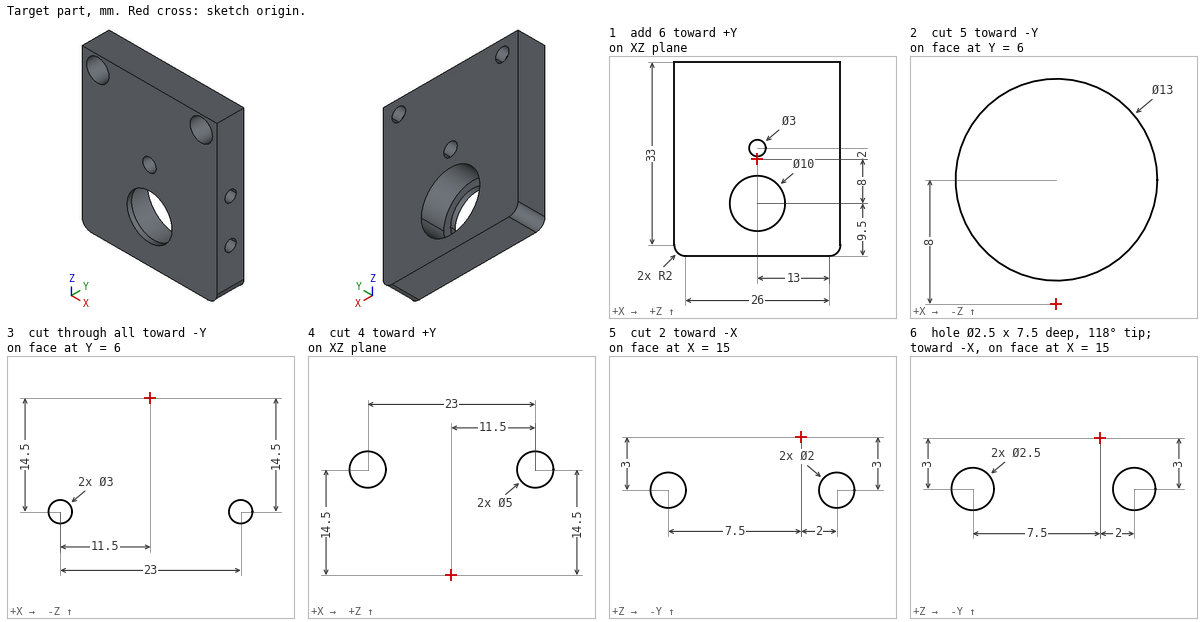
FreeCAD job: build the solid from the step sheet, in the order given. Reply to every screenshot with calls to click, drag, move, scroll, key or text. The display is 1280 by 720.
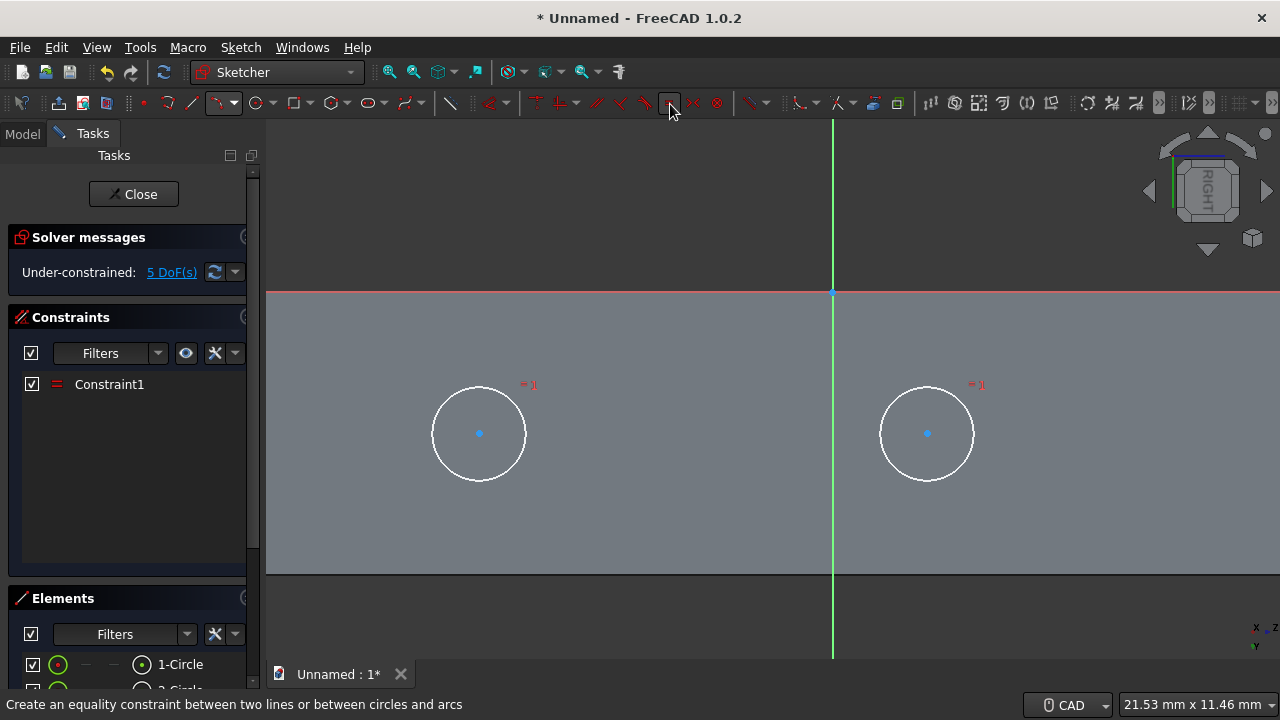
click(490, 104)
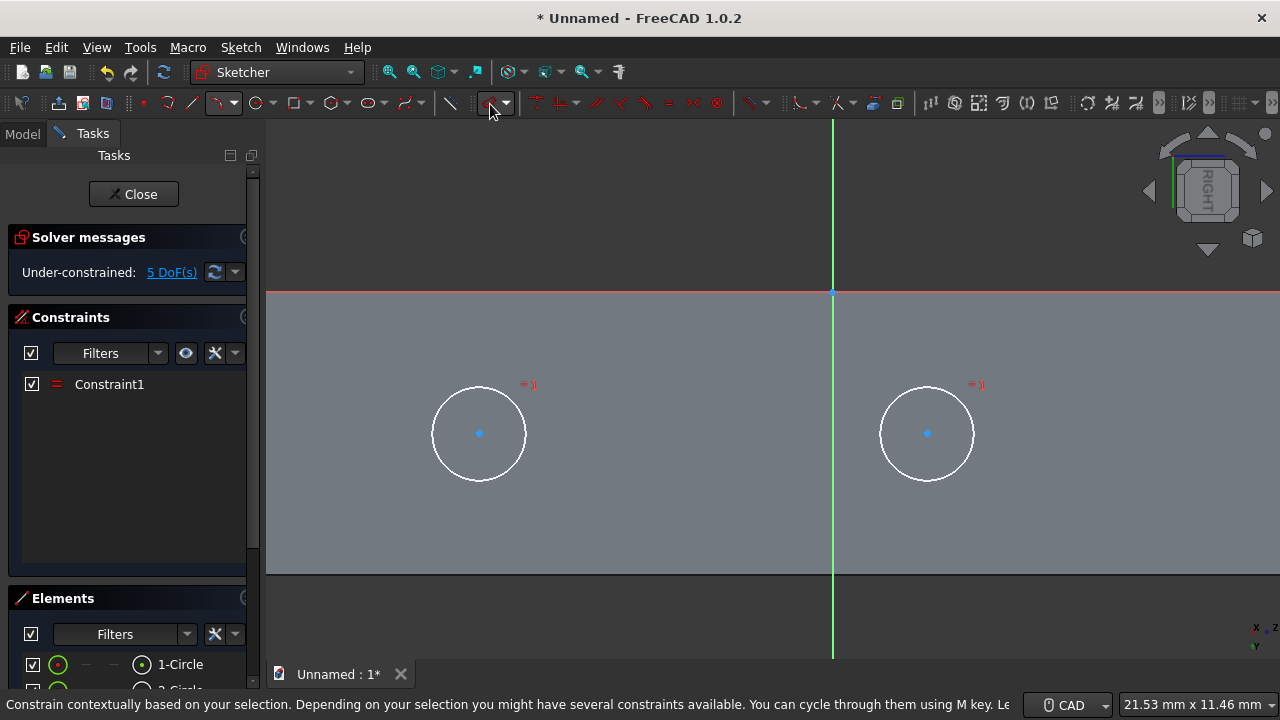
click(960, 401)
click(983, 378)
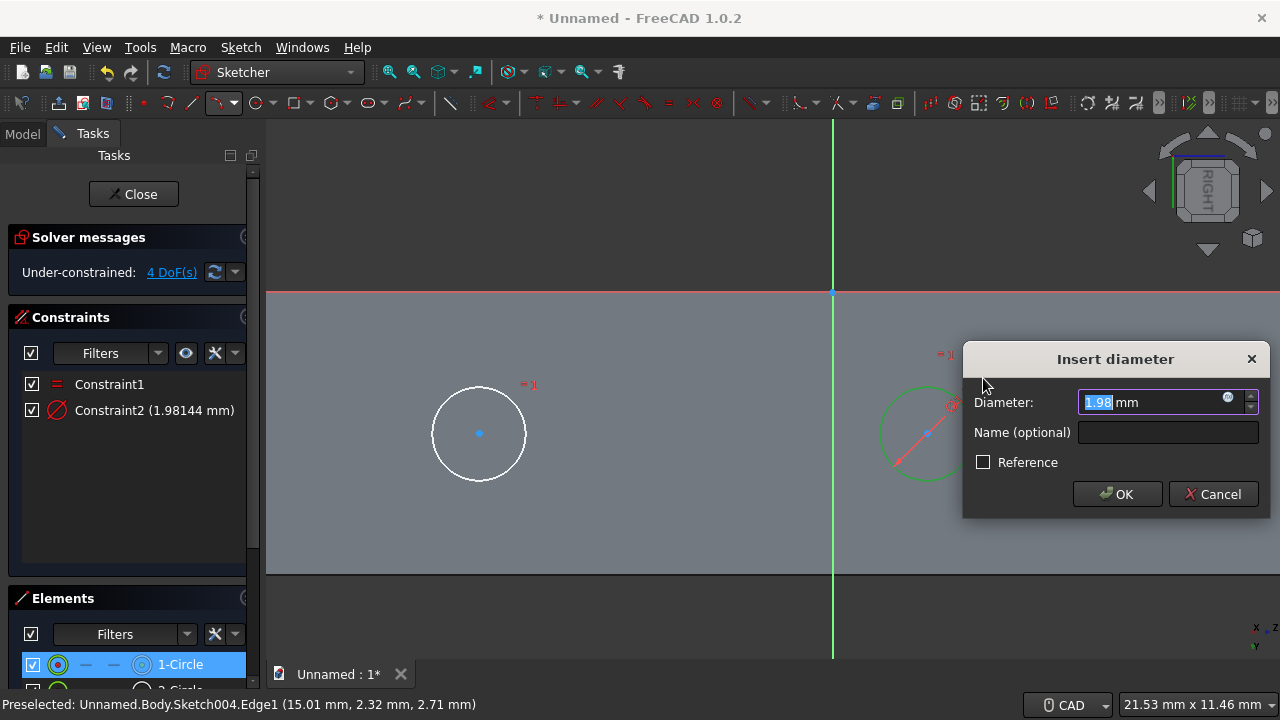
text(2)
key(Return)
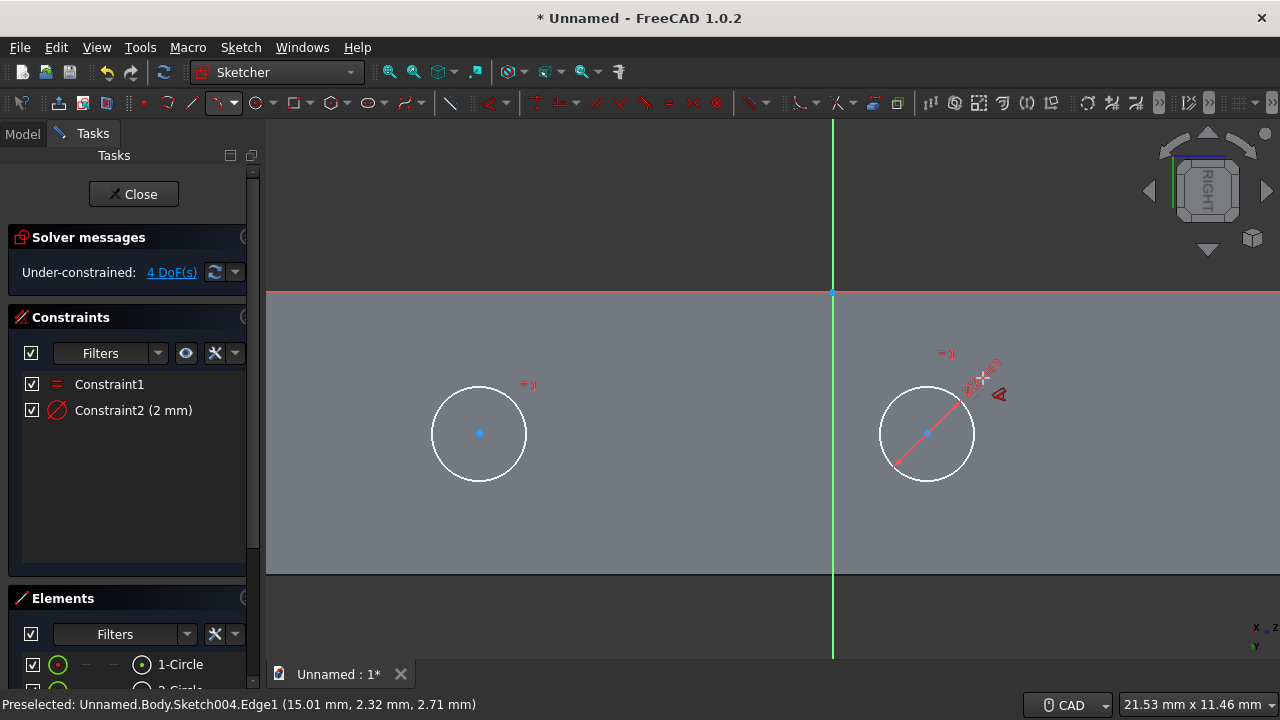
click(927, 434)
click(880, 258)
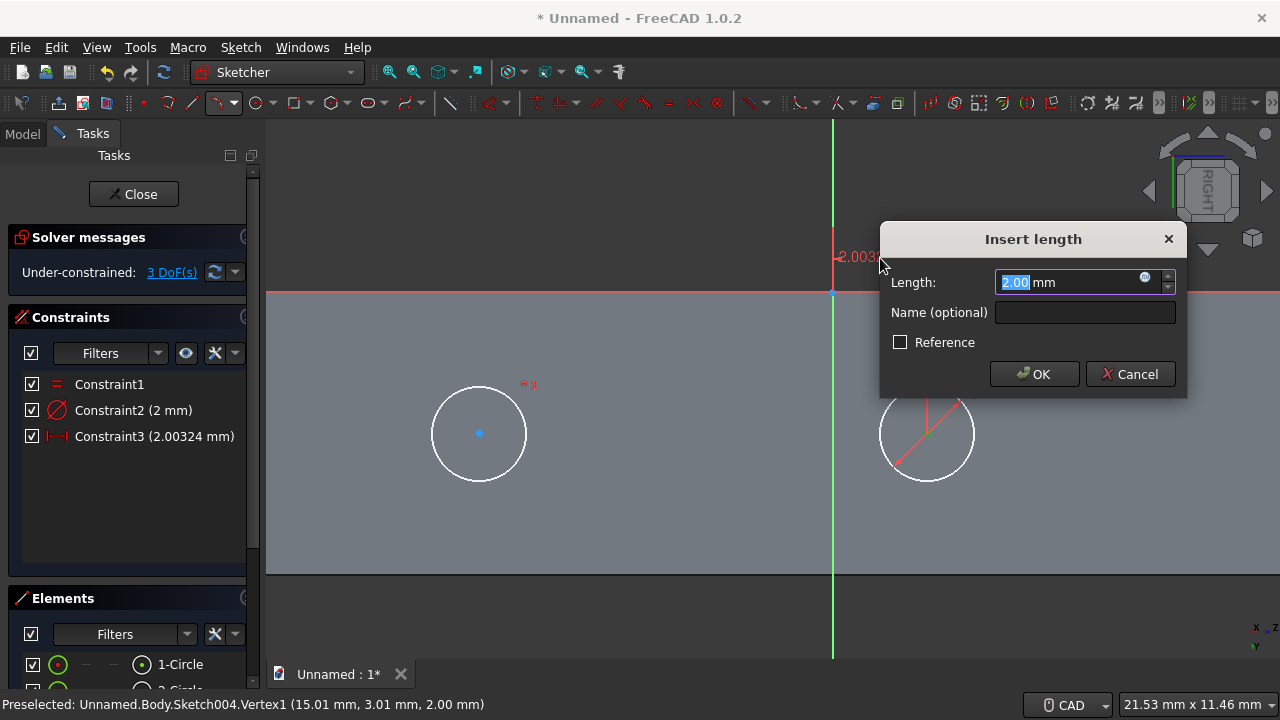
text(2)
key(Return)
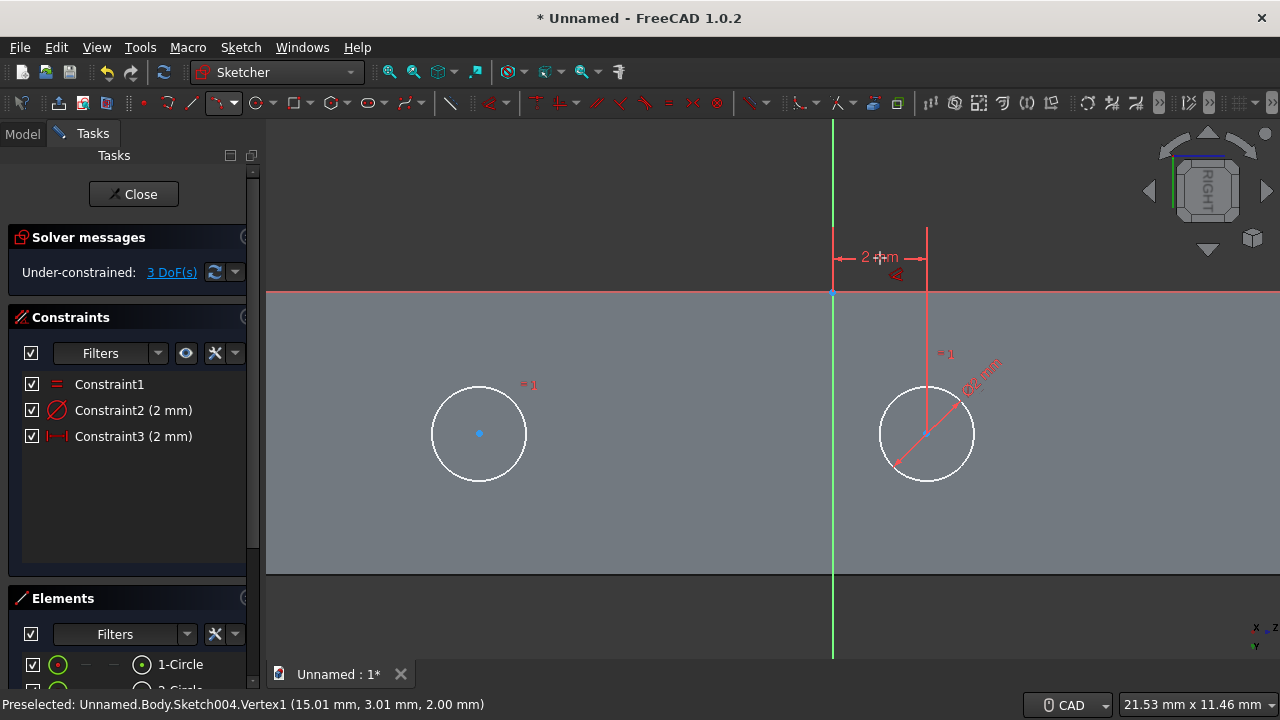
click(927, 434)
click(961, 330)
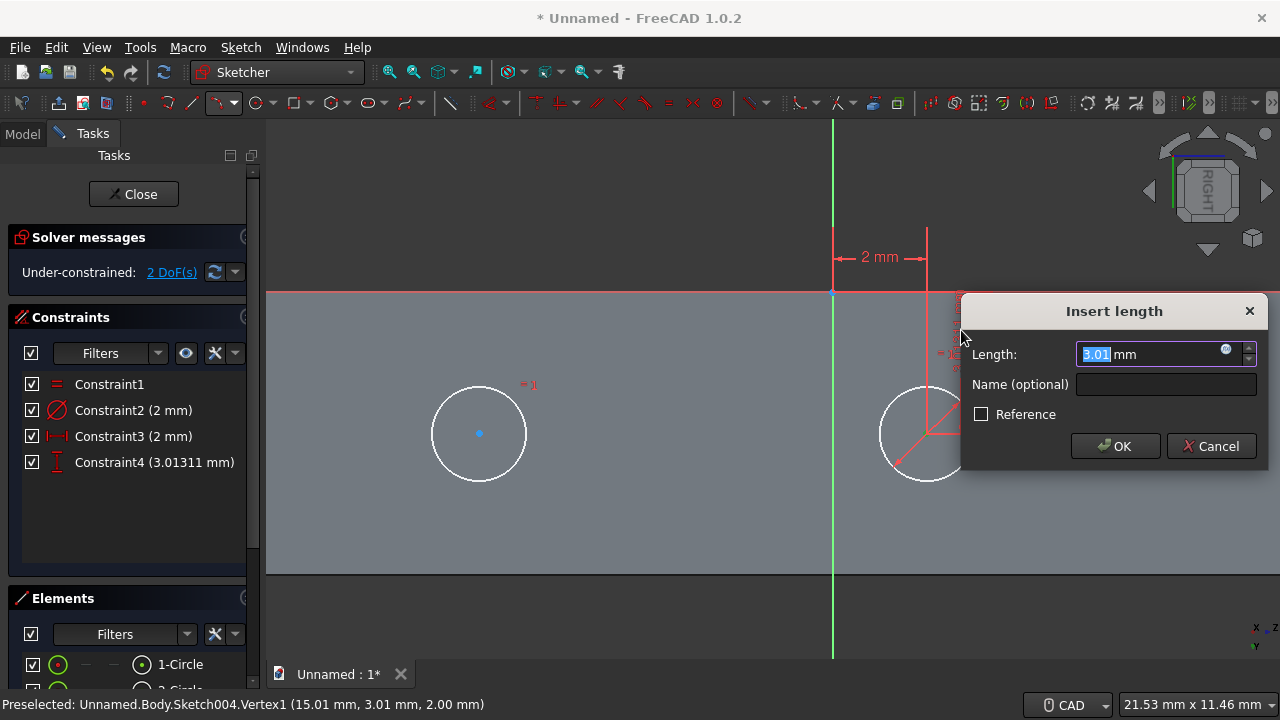
text(3)
key(Return)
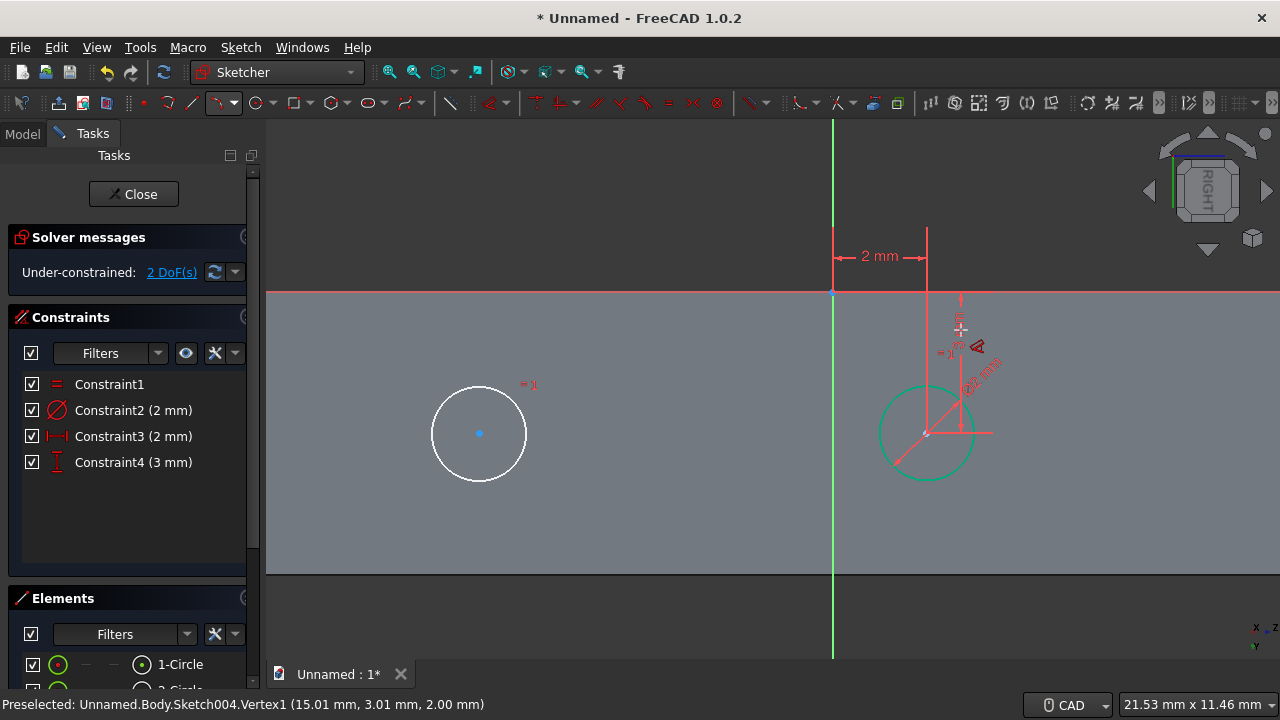
click(479, 434)
click(445, 363)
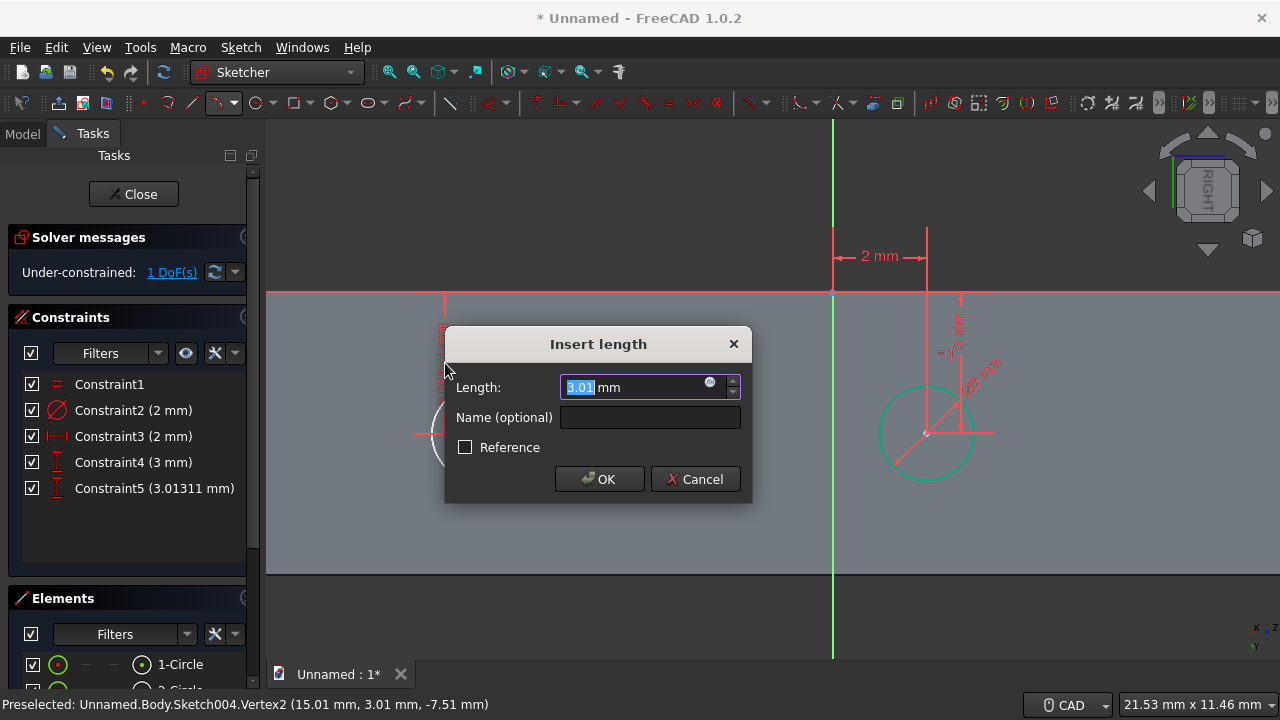
text(3)
key(Return)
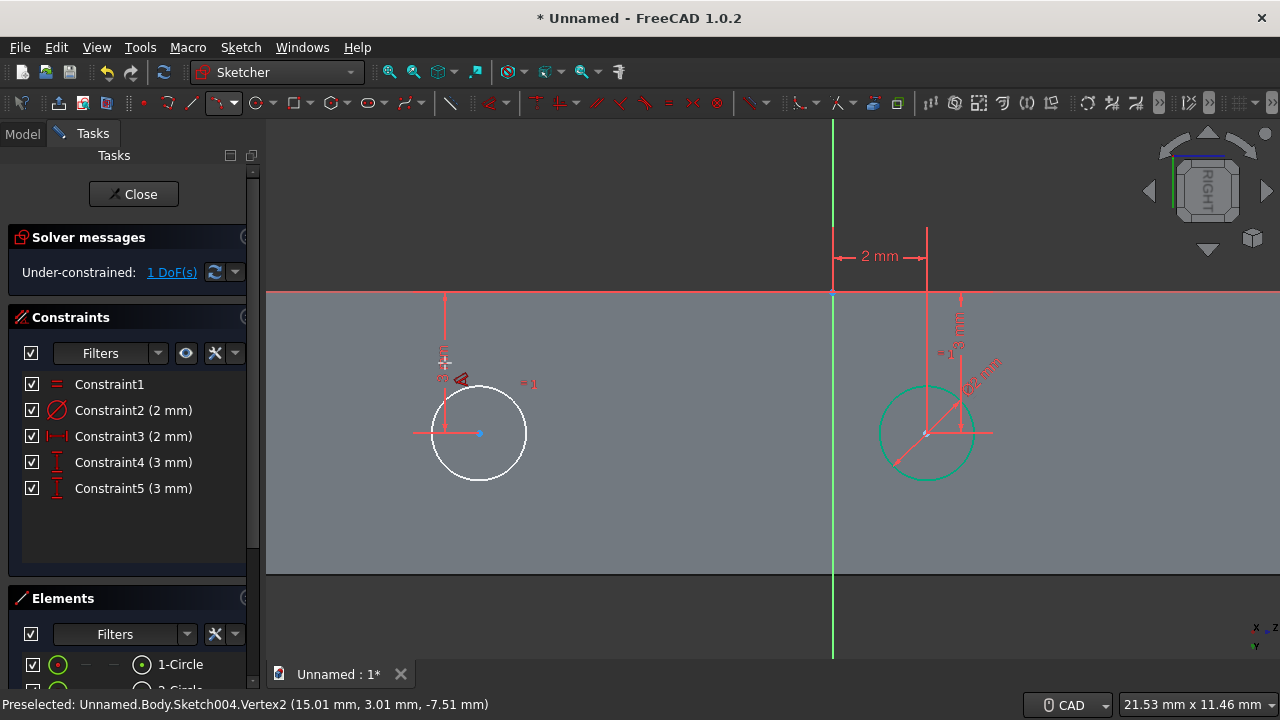
click(479, 433)
click(656, 258)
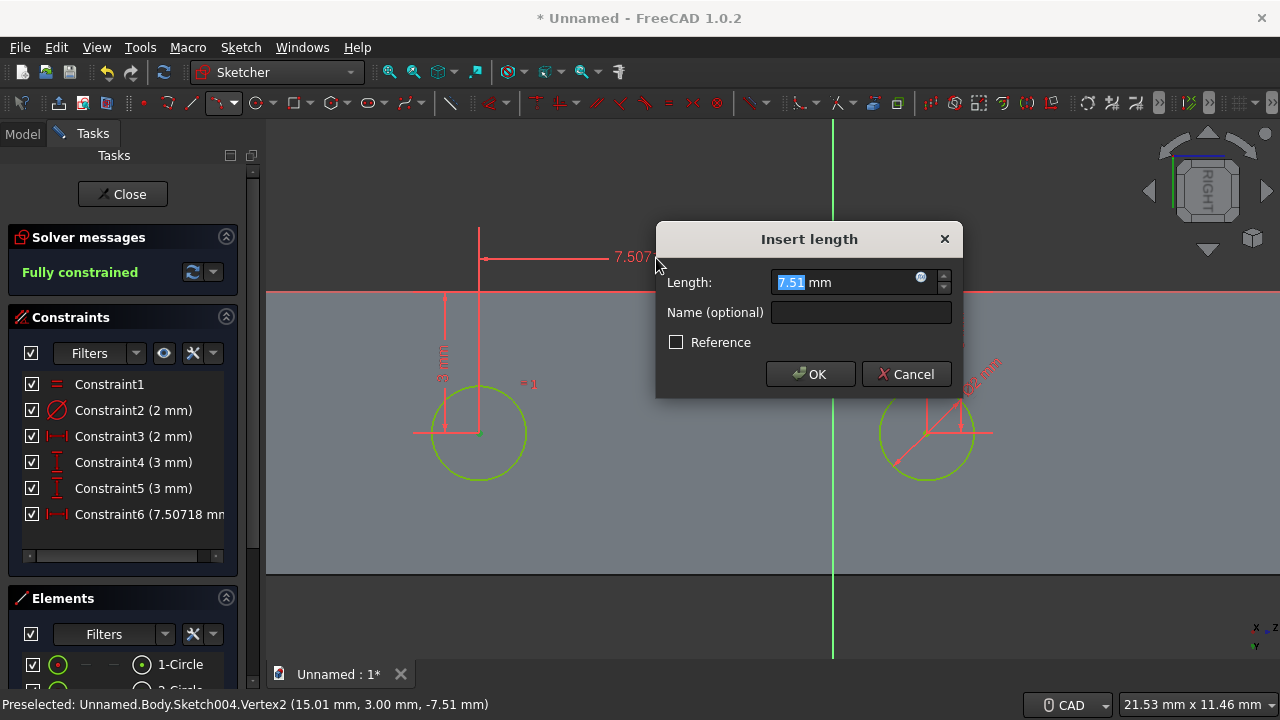
text(7.5)
key(Return)
key(Escape)